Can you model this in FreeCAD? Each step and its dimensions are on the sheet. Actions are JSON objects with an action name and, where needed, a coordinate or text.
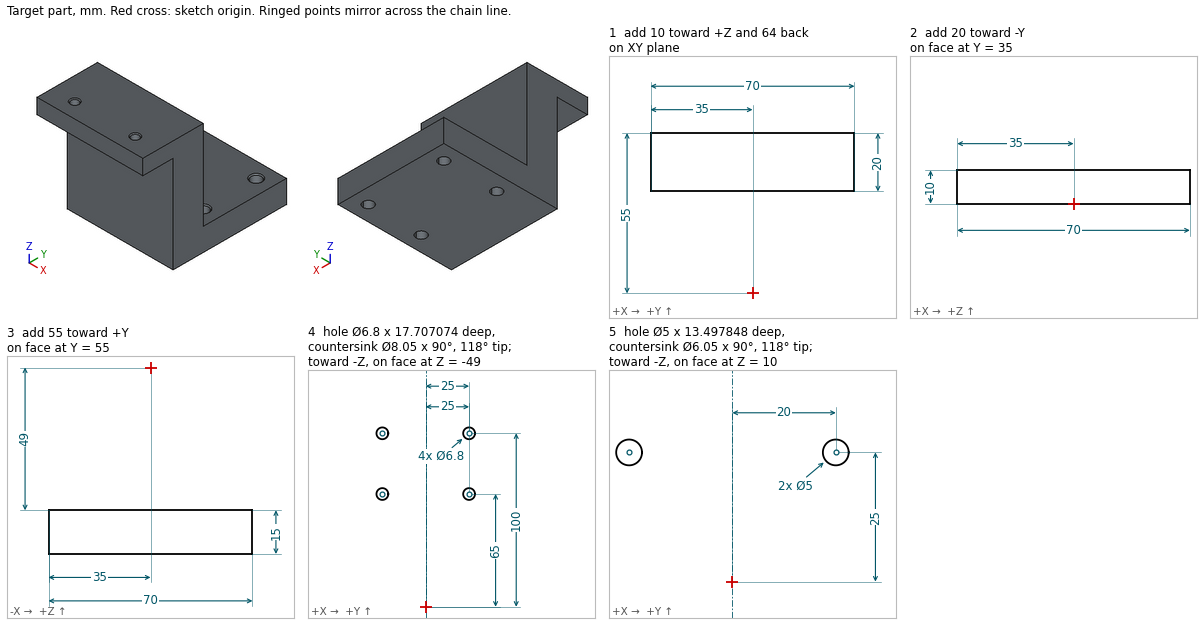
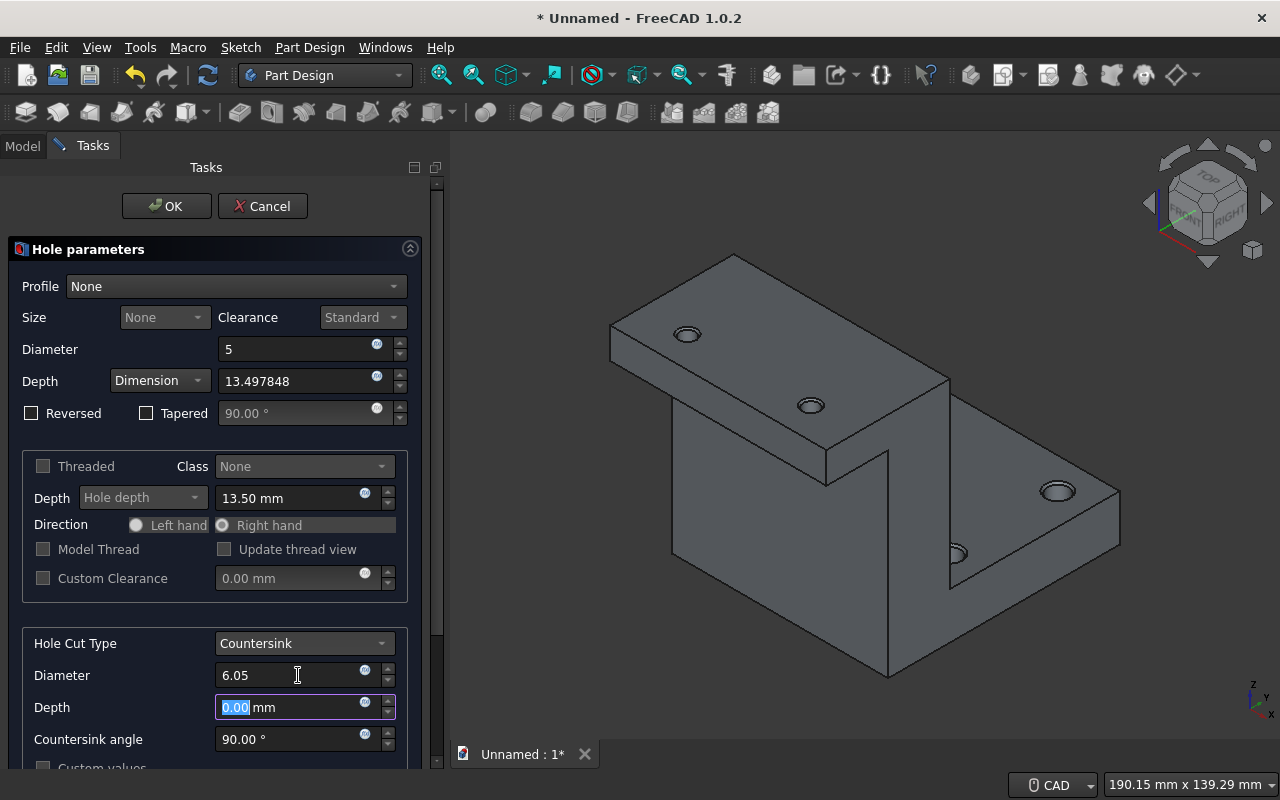
{"action": "left_click", "coordinate": [167, 206]}